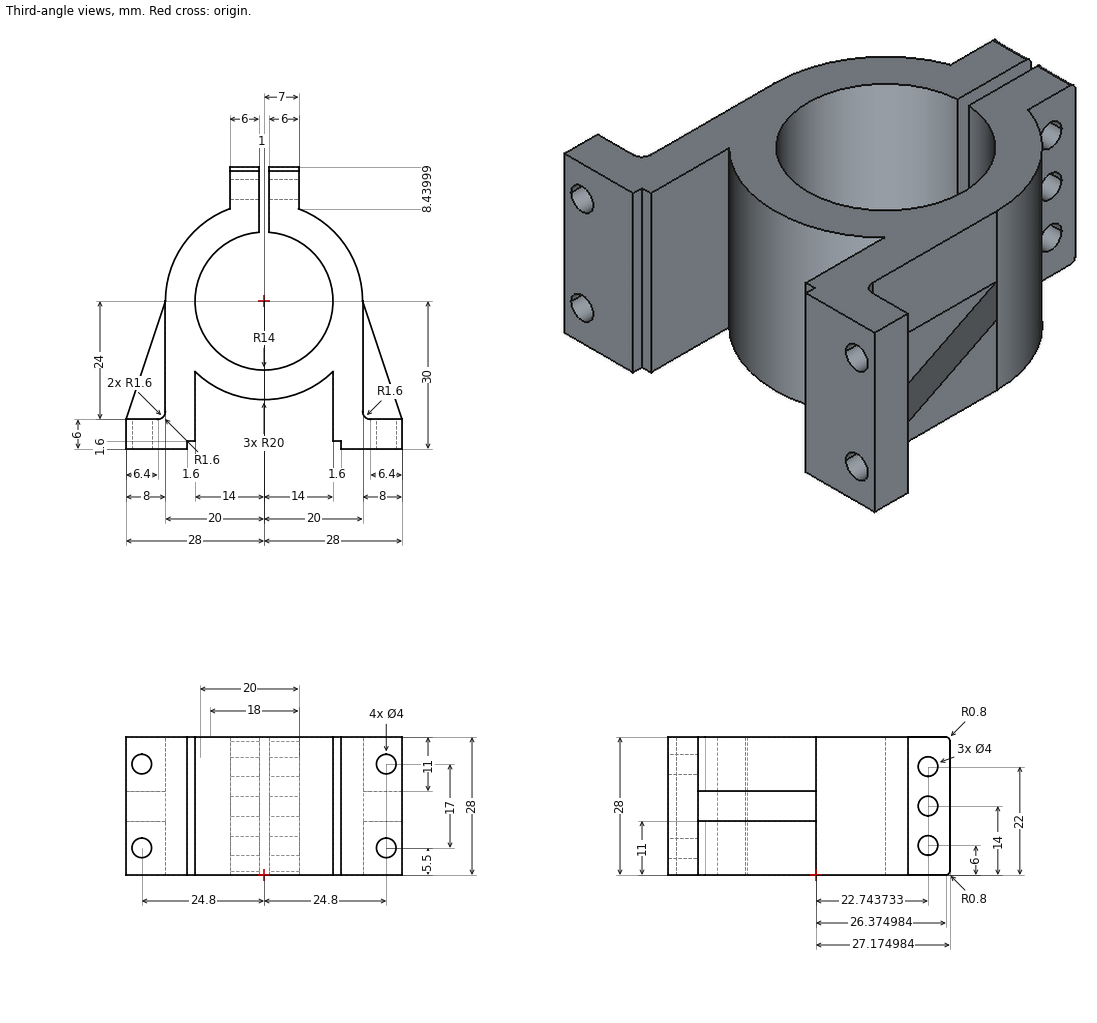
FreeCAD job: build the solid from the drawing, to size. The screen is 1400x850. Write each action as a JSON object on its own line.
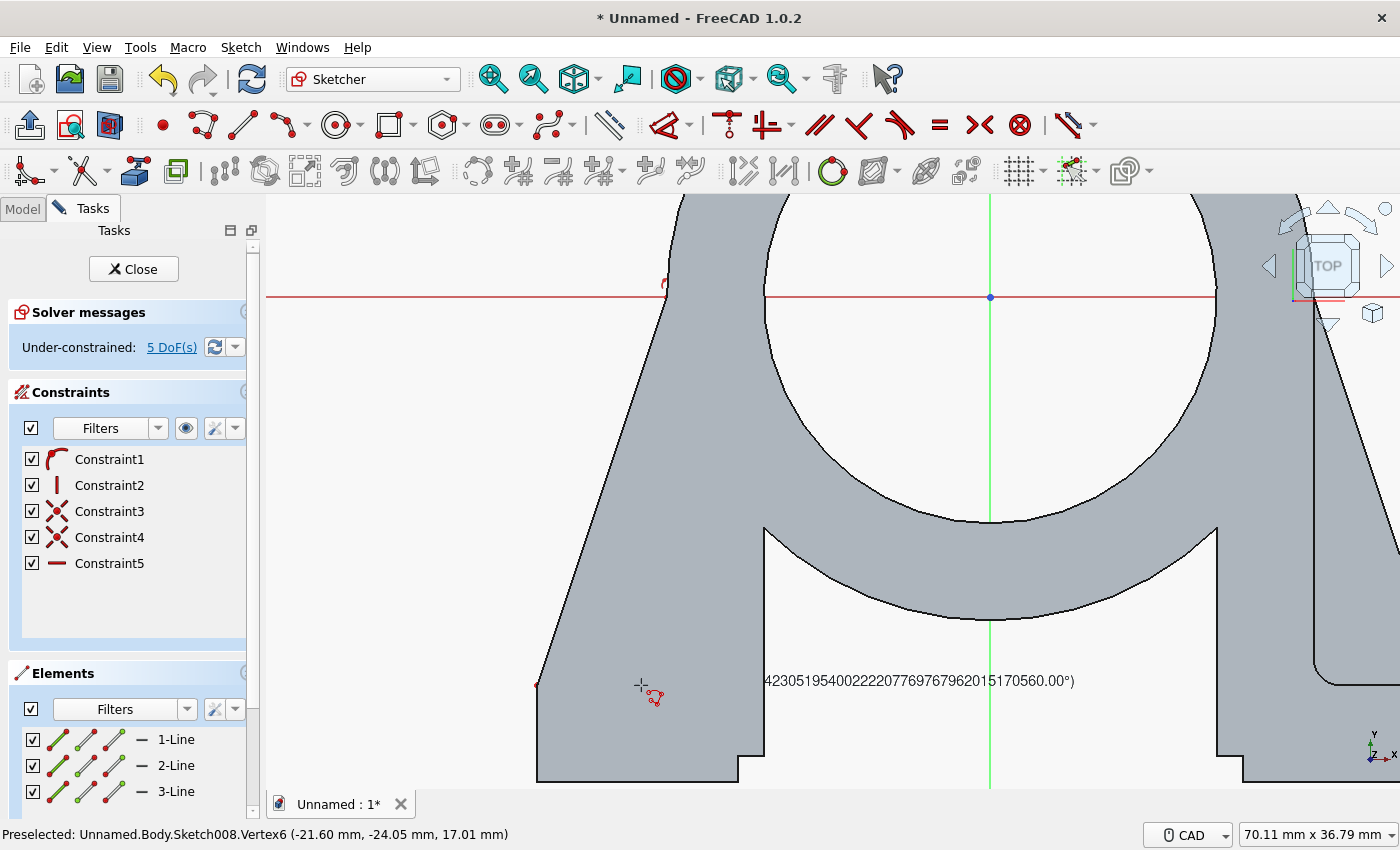
{"action": "left_click", "coordinate": [284, 126]}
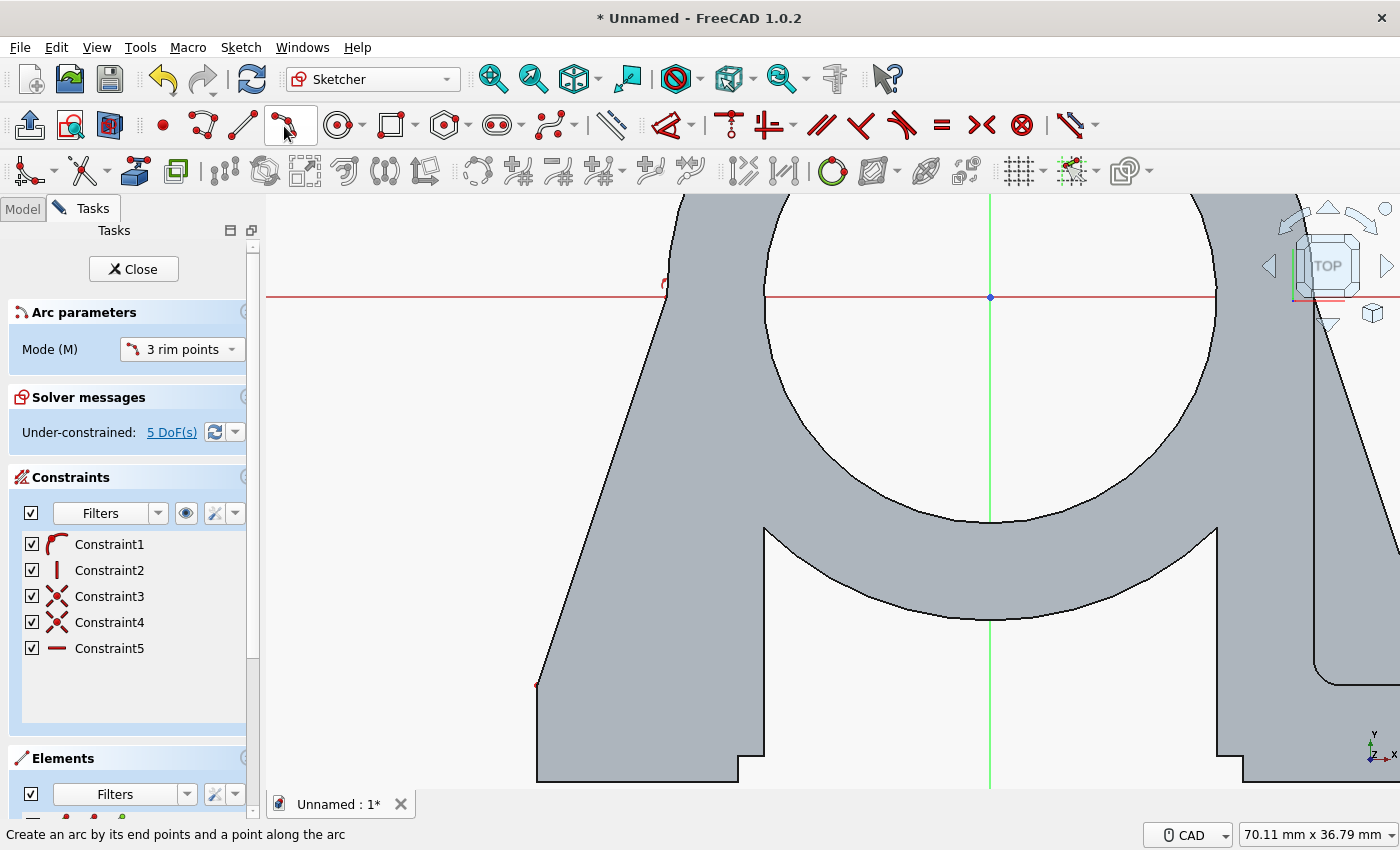
{"action": "left_click", "coordinate": [641, 686]}
{"action": "left_click", "coordinate": [667, 660]}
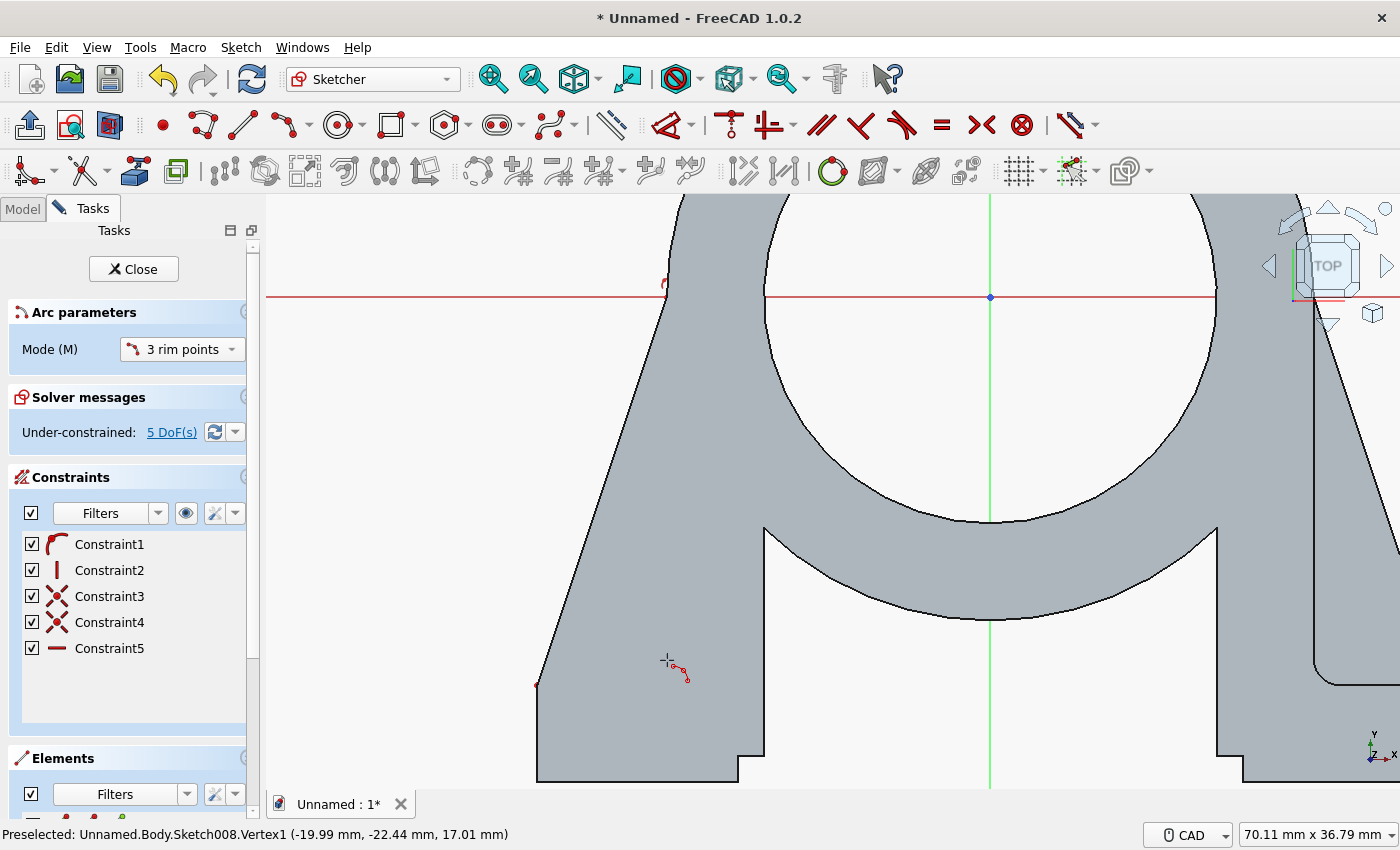
{"action": "scroll", "coordinate": [659, 678], "scroll_direction": "up", "scroll_amount": 4}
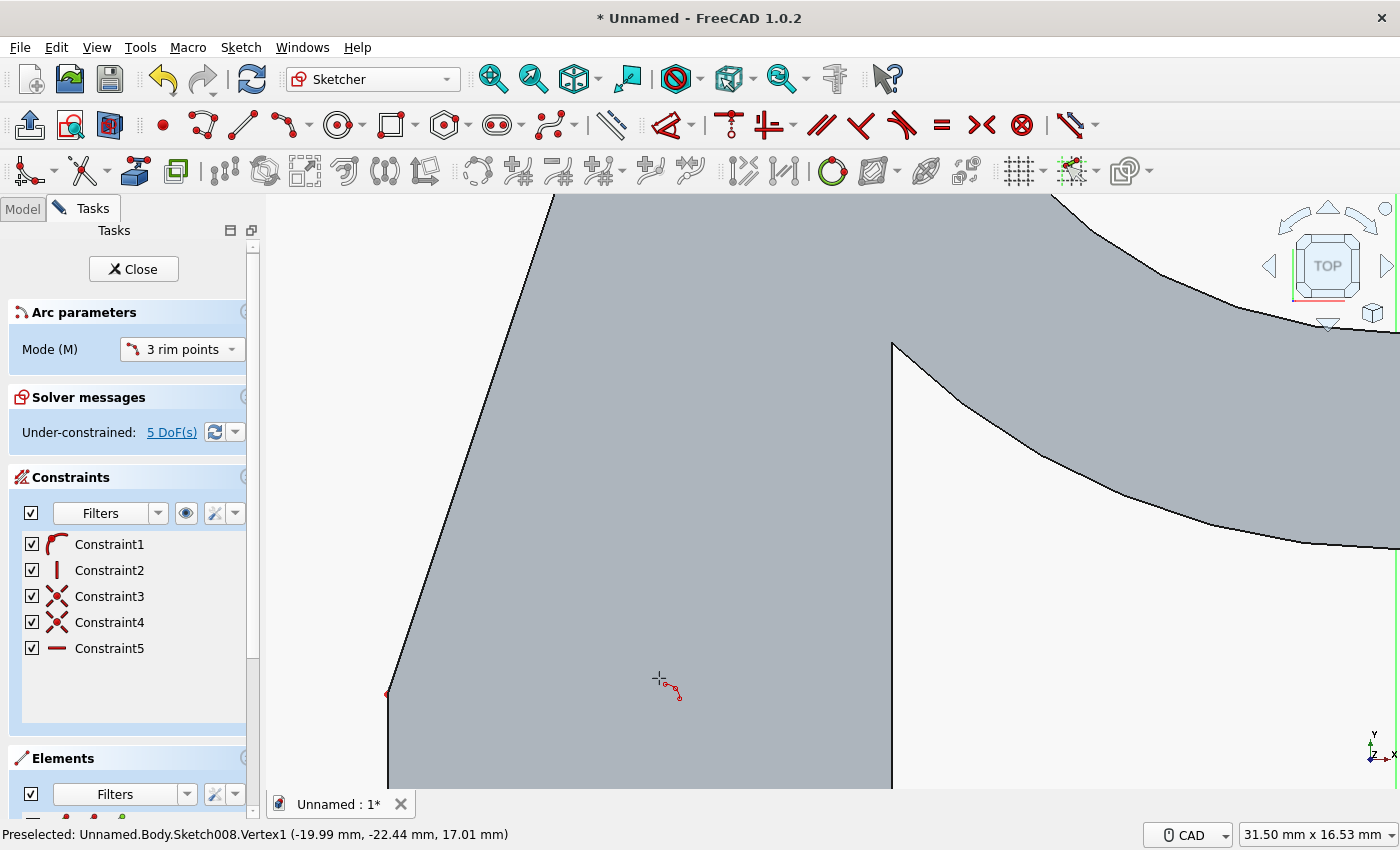
{"action": "left_click", "coordinate": [659, 676]}
{"action": "key", "text": "Escape"}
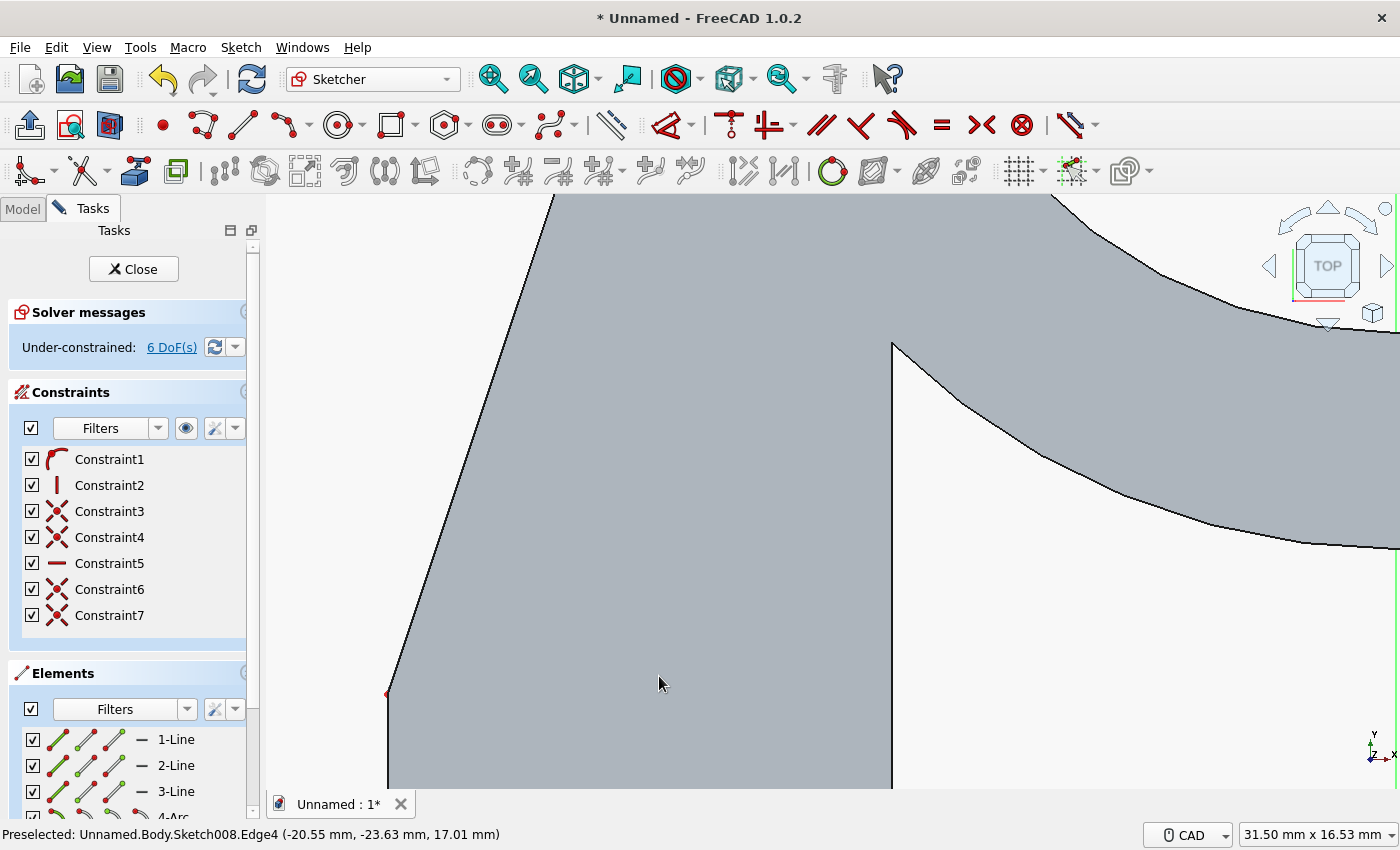
{"action": "left_click", "coordinate": [676, 395]}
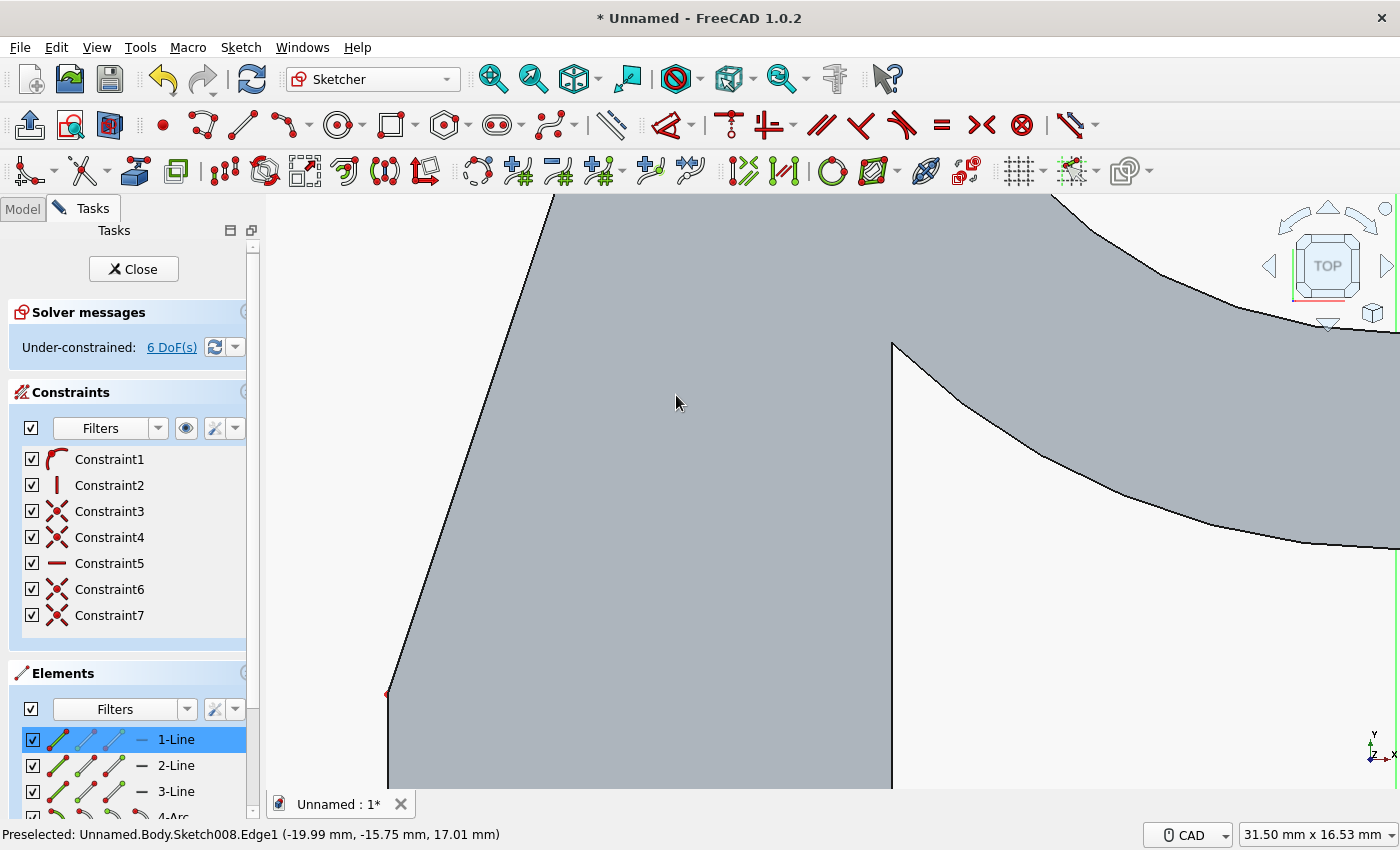
{"action": "left_click", "coordinate": [644, 688]}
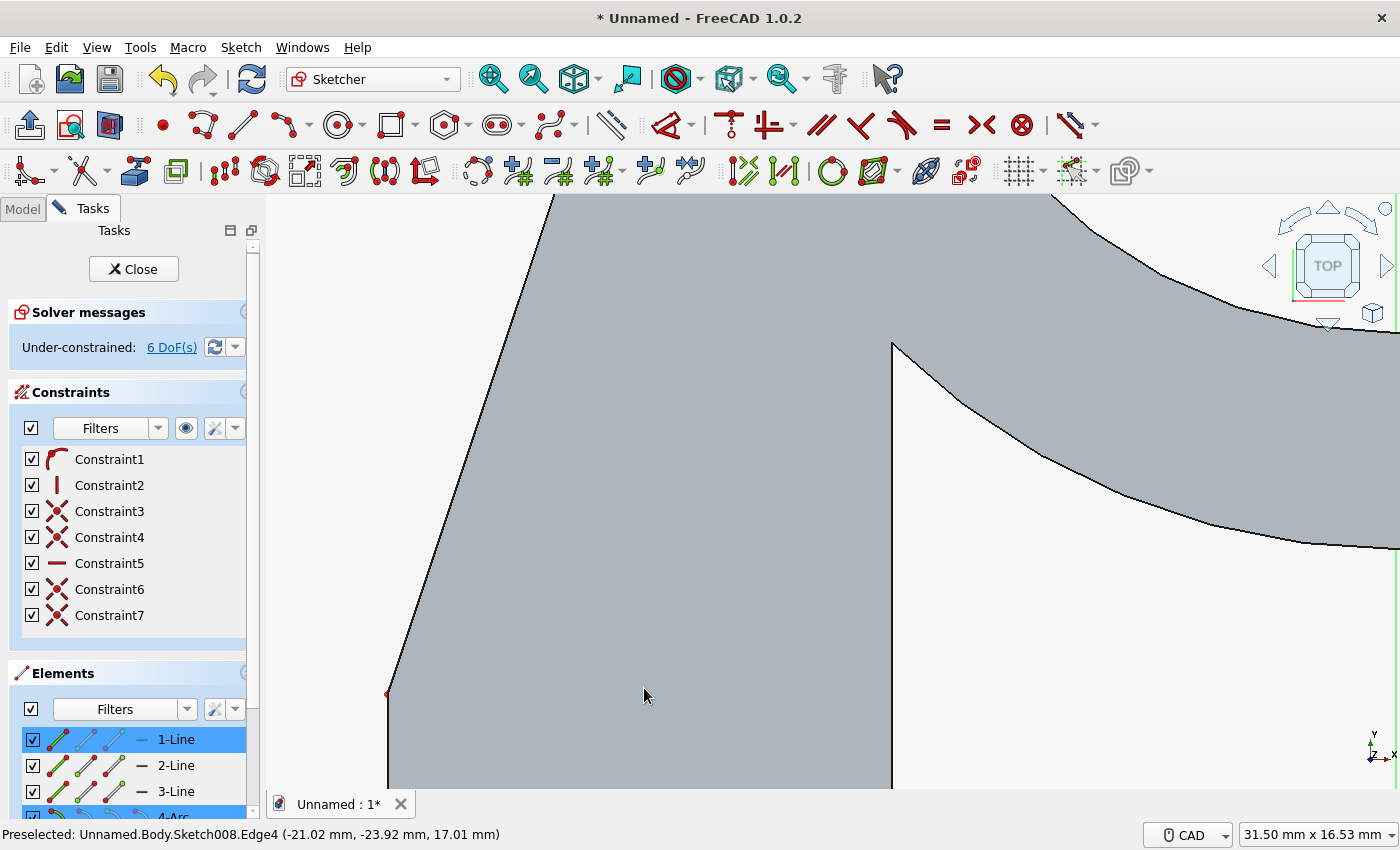
{"action": "left_click", "coordinate": [902, 126]}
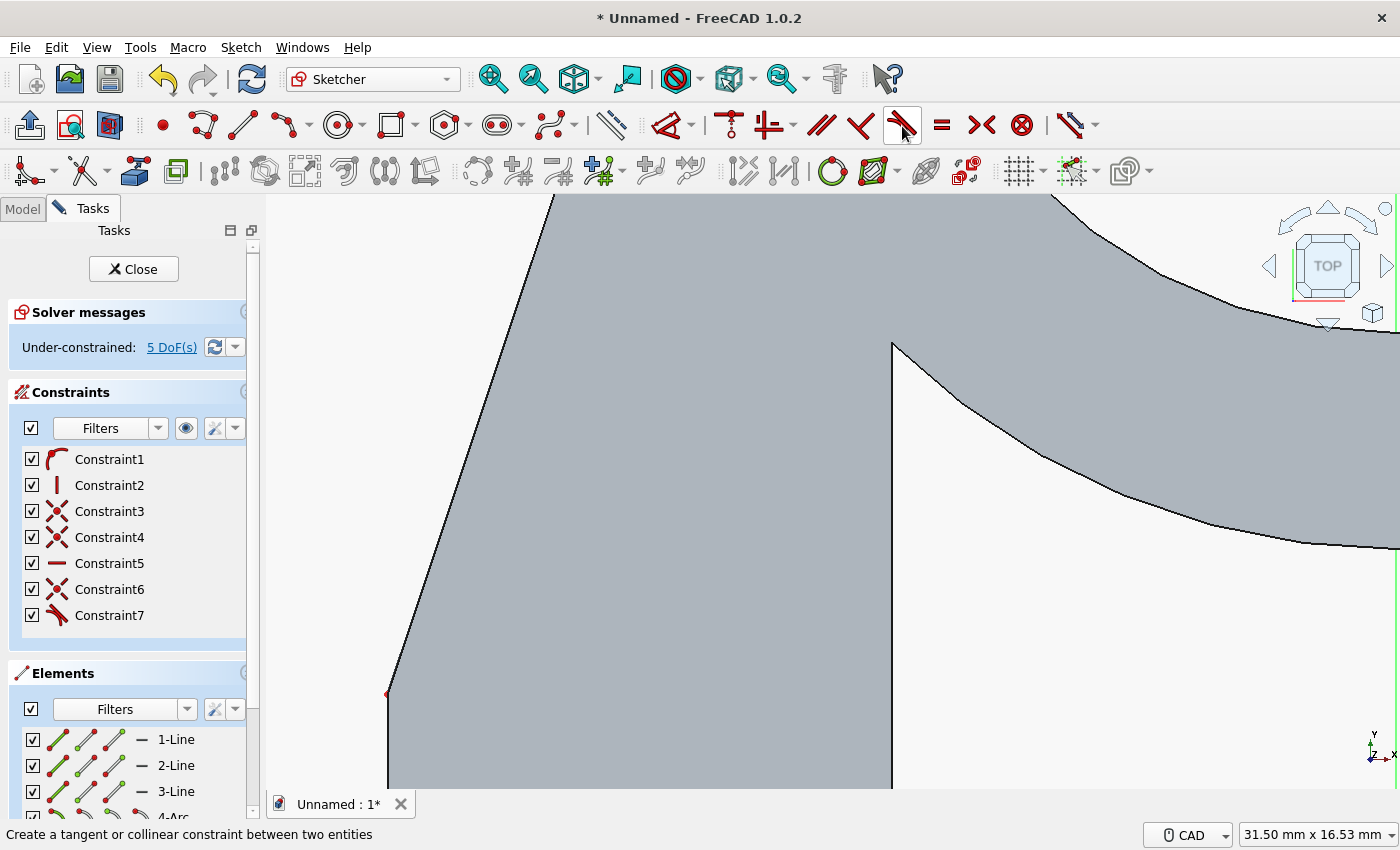
{"action": "left_click", "coordinate": [456, 695]}